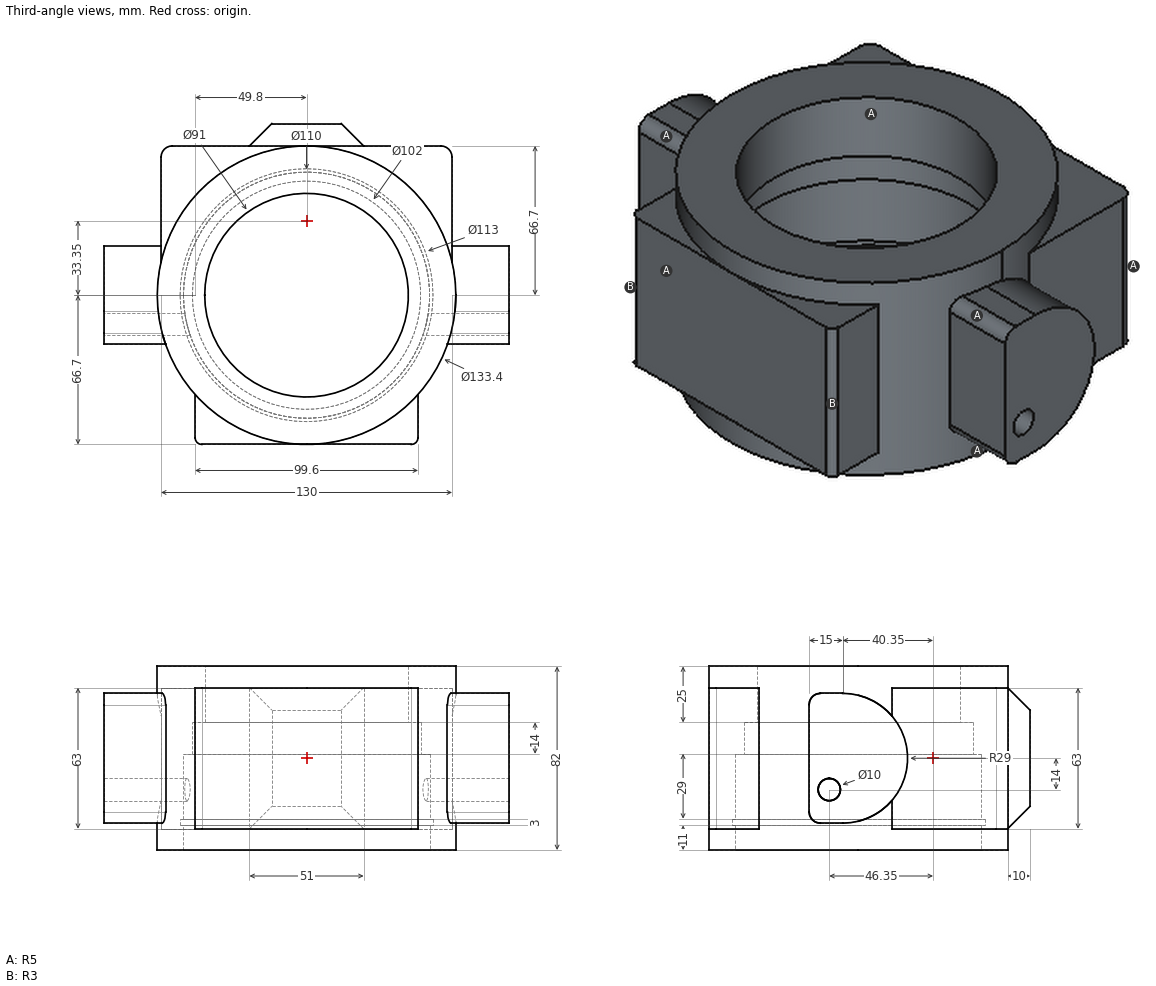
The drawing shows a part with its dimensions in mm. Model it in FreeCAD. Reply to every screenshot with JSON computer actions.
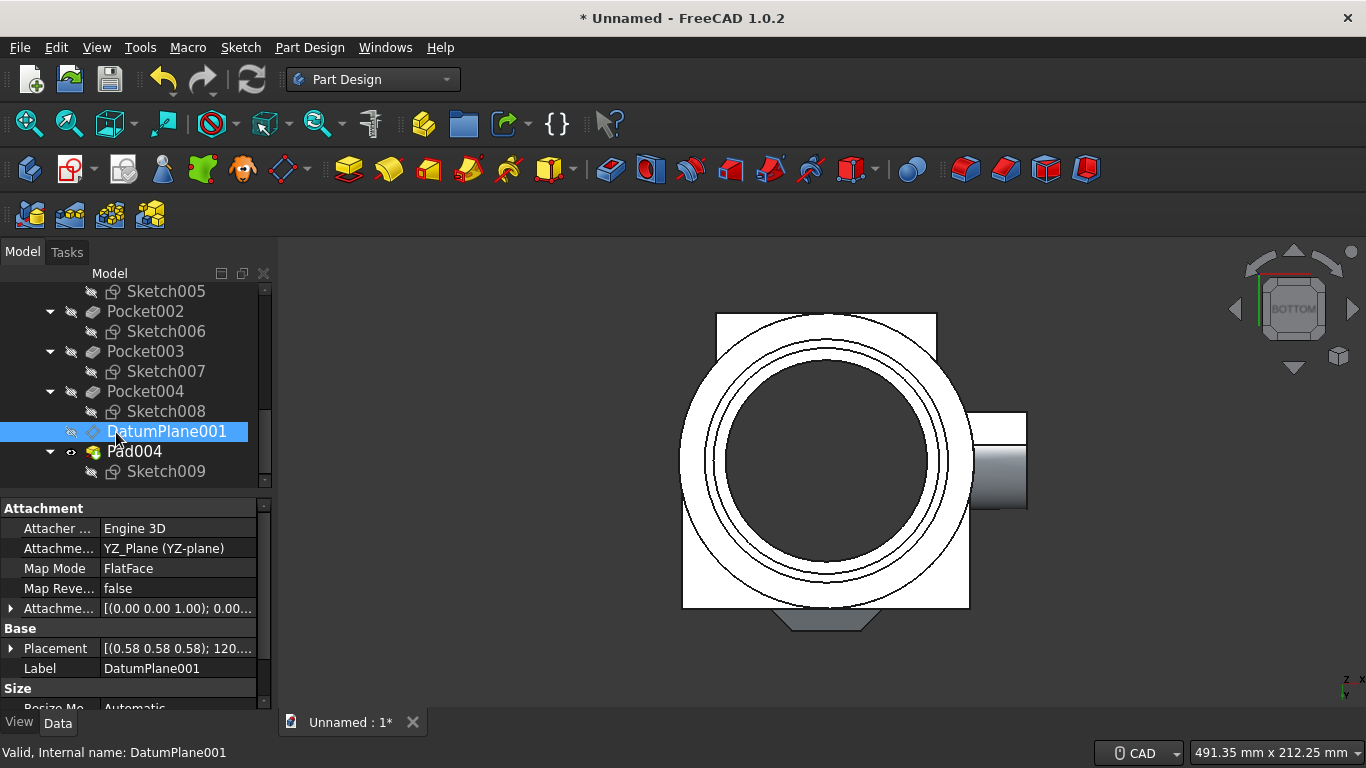
{"action": "scroll", "coordinate": [160, 387], "scroll_direction": "down", "scroll_amount": 3}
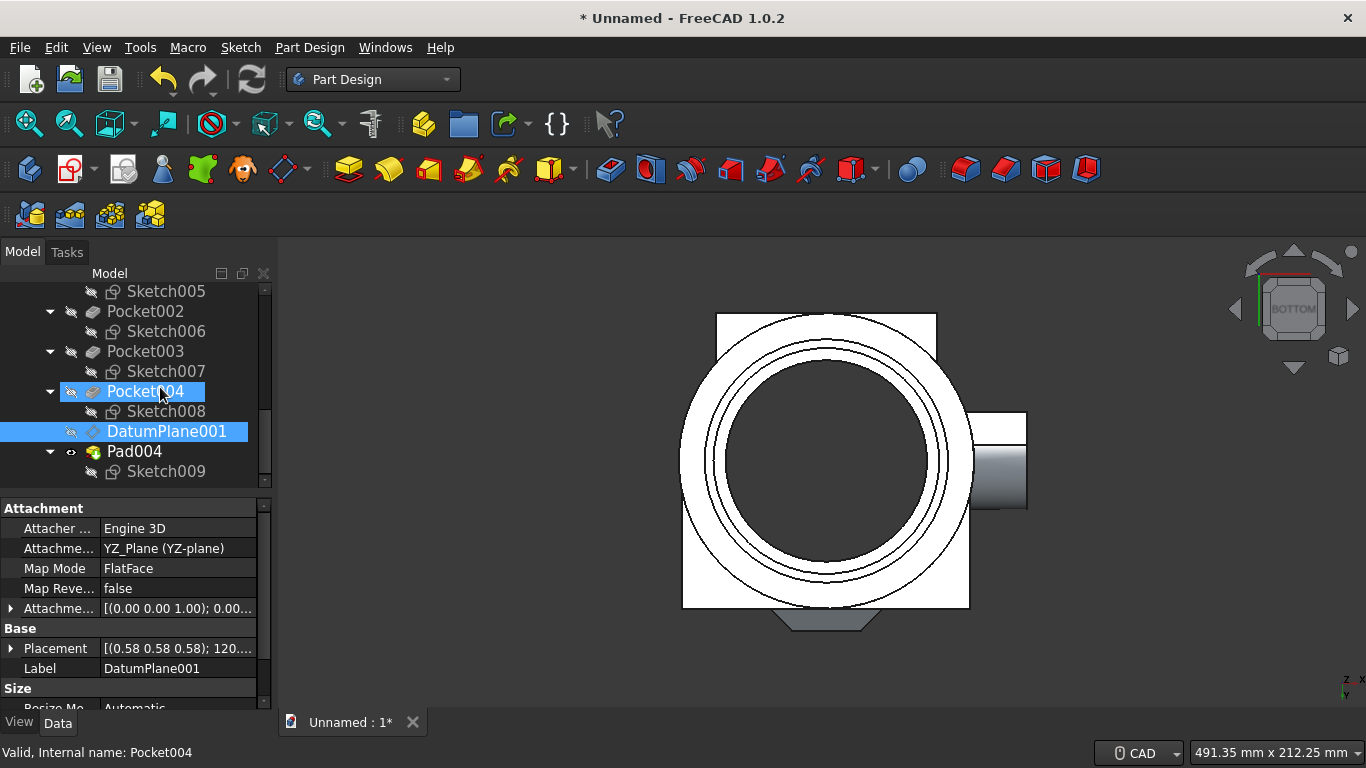
{"action": "scroll", "coordinate": [160, 387], "scroll_direction": "up", "scroll_amount": 15}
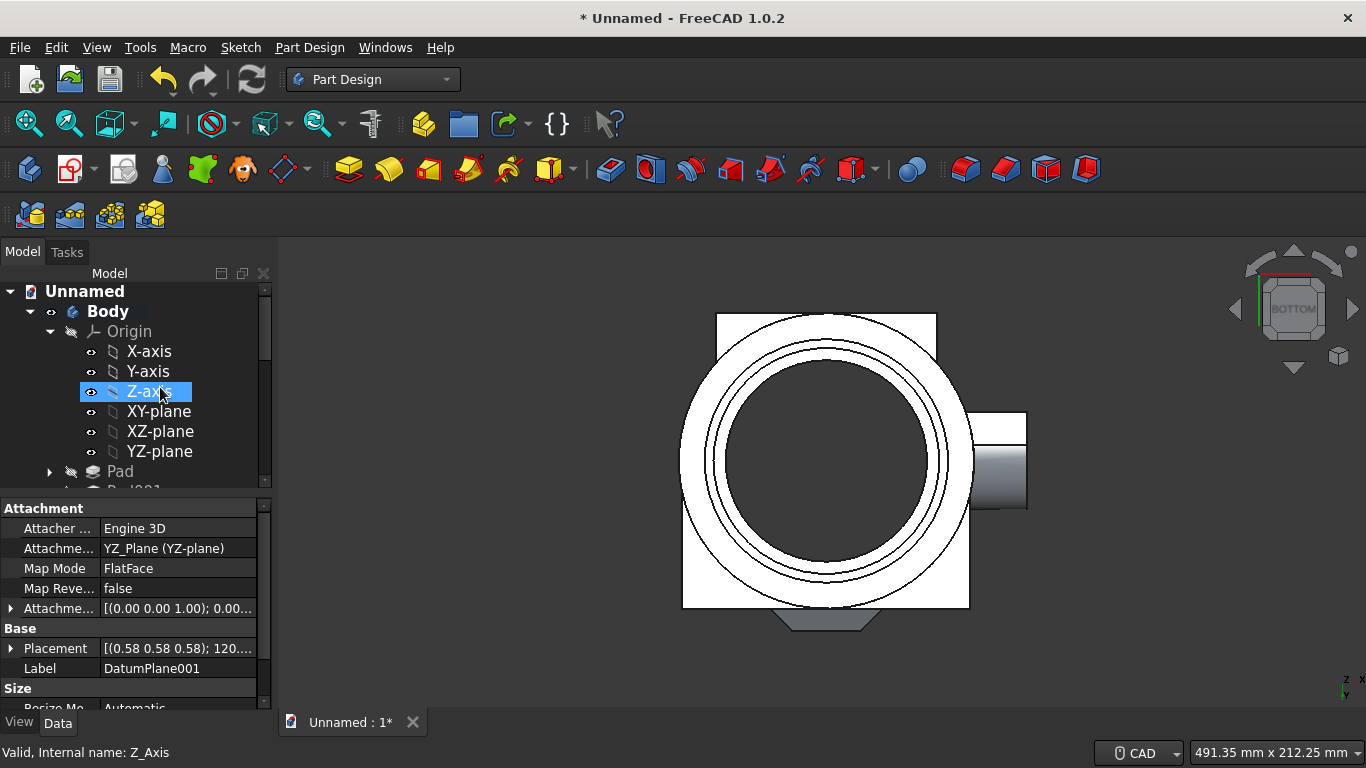
{"action": "left_click", "coordinate": [136, 452]}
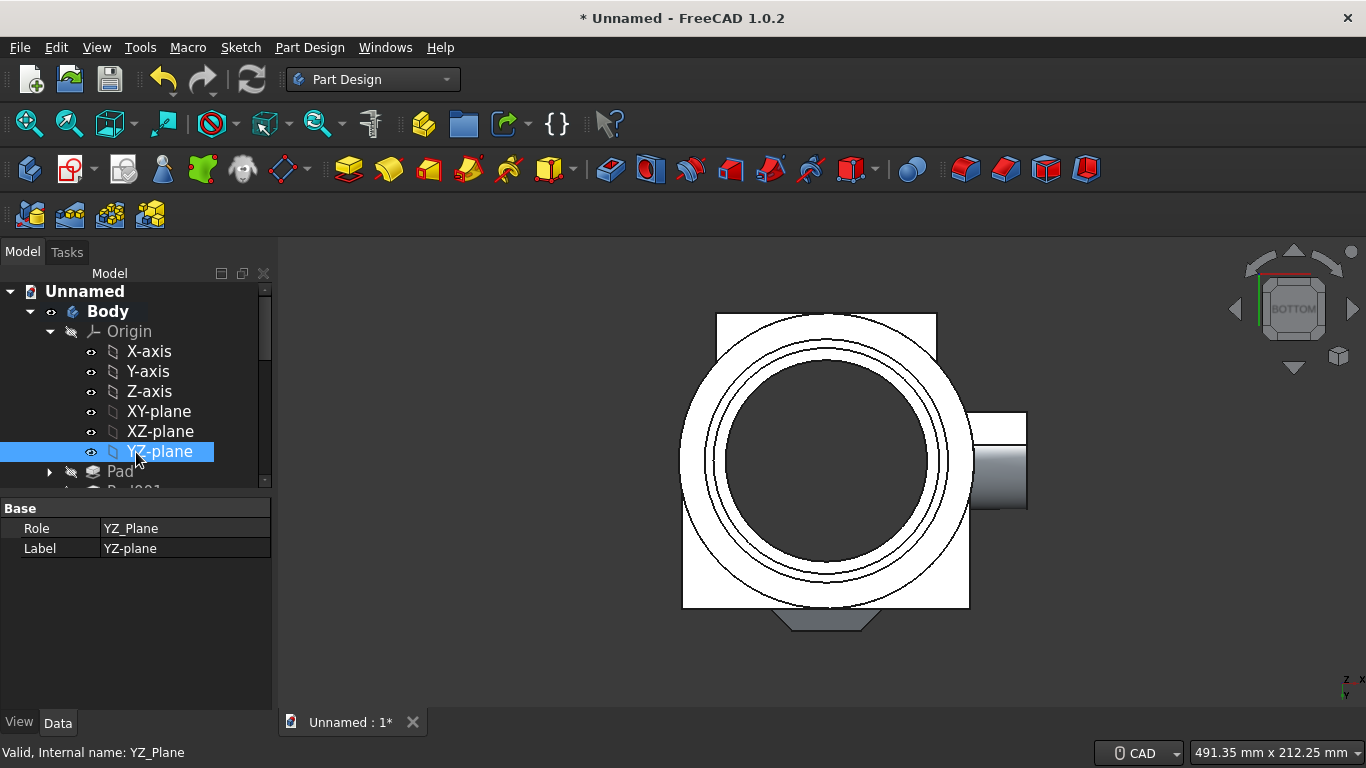
{"action": "left_click", "coordinate": [284, 170]}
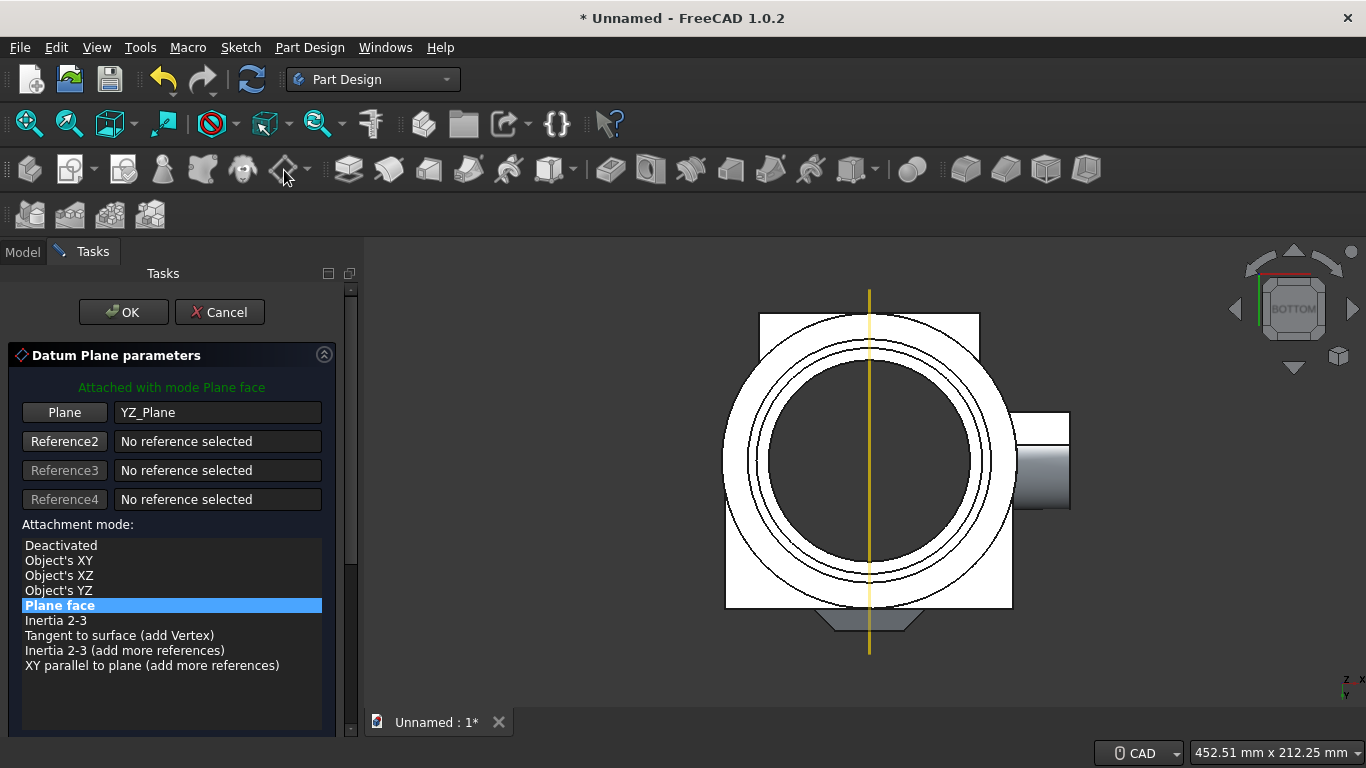
{"action": "scroll", "coordinate": [351, 510], "scroll_direction": "down", "scroll_amount": 3}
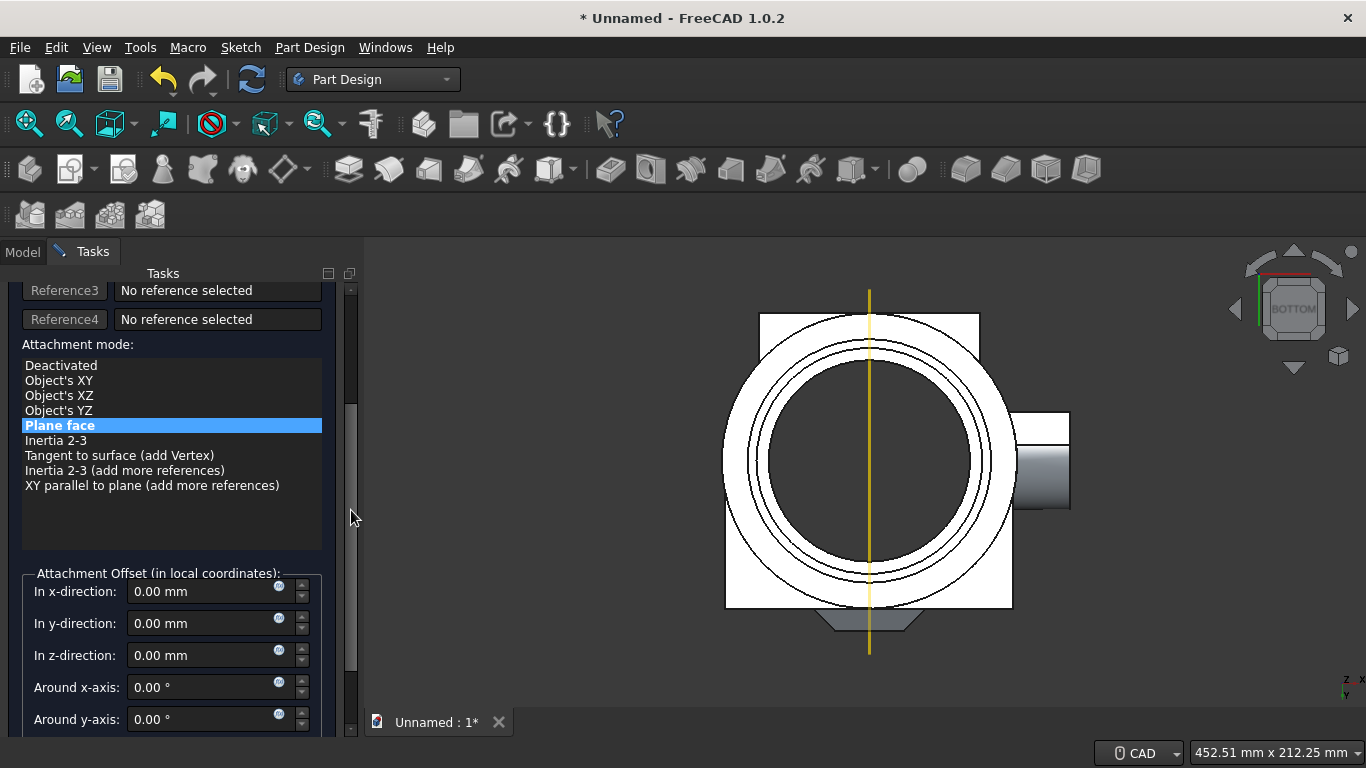
{"action": "triple_click", "coordinate": [210, 655]}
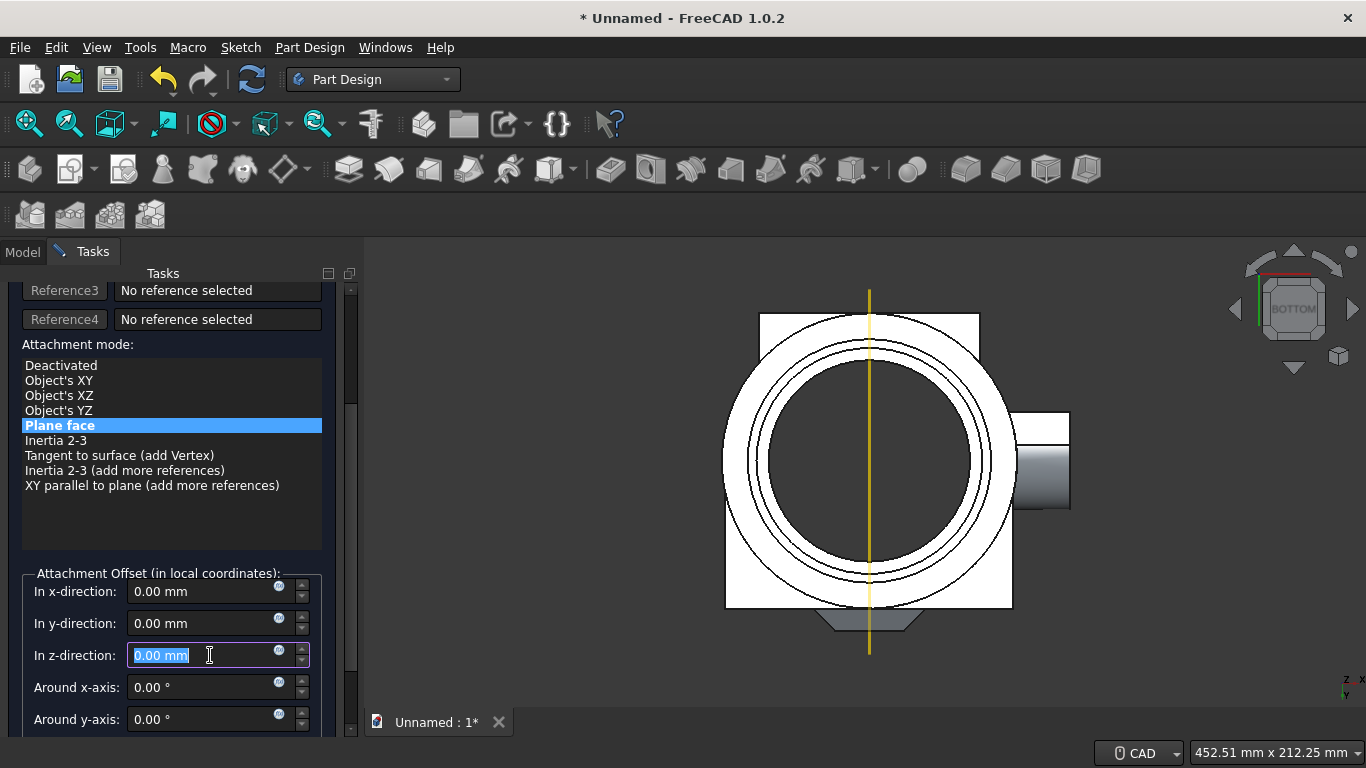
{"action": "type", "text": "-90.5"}
{"action": "key", "text": "Tab"}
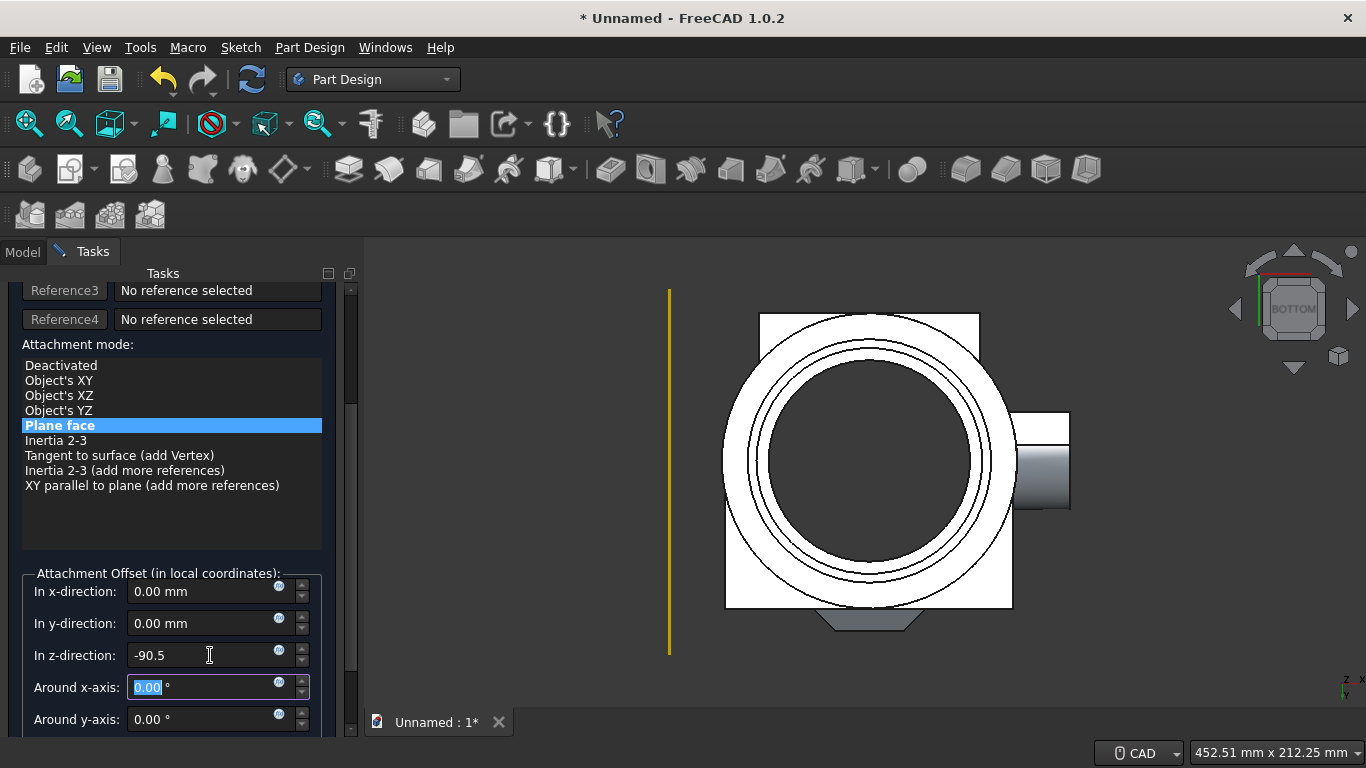
{"action": "scroll", "coordinate": [351, 510], "scroll_direction": "up", "scroll_amount": 4}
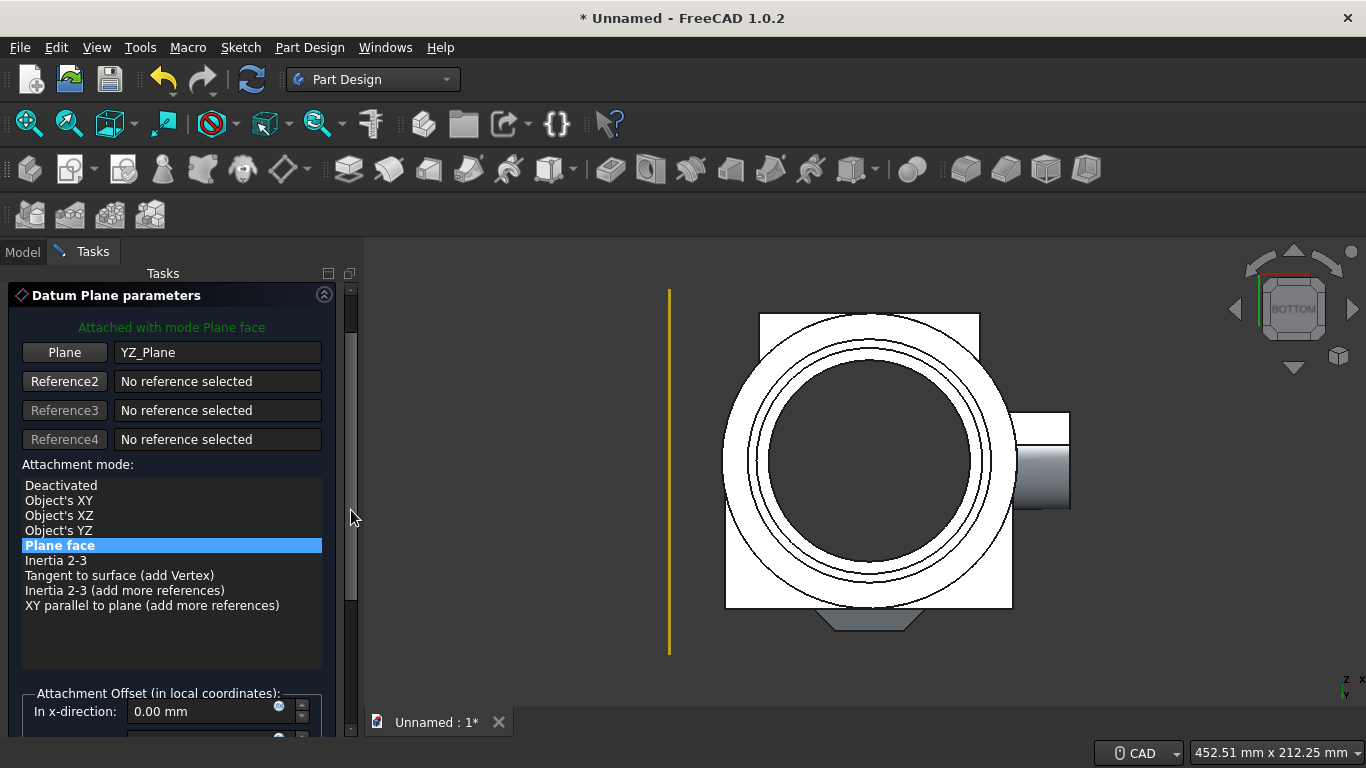
{"action": "left_click", "coordinate": [124, 312]}